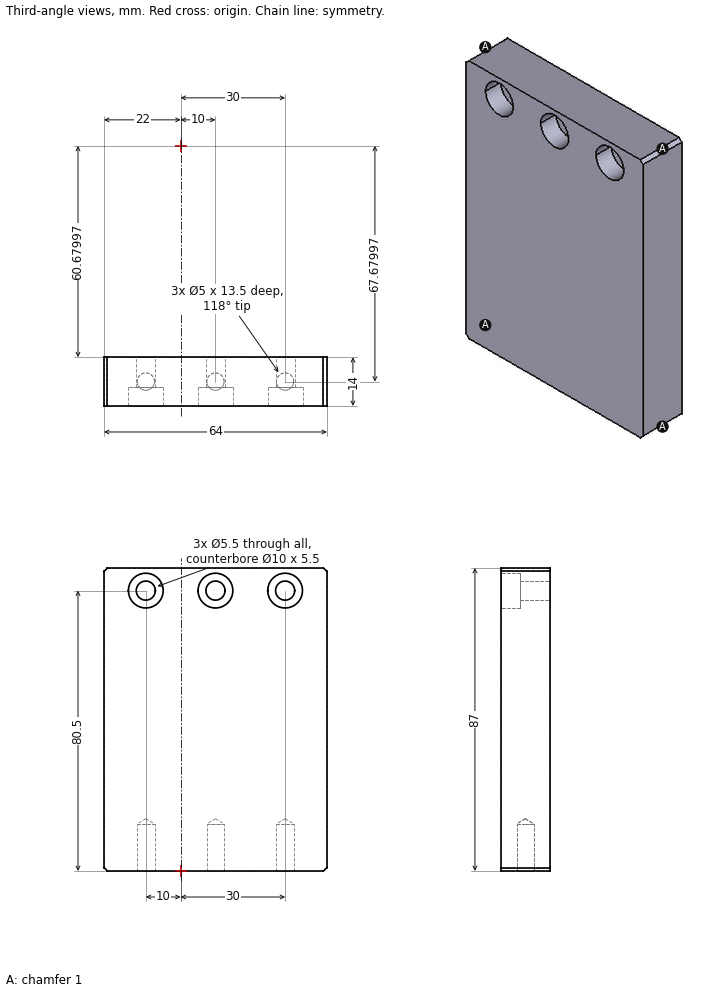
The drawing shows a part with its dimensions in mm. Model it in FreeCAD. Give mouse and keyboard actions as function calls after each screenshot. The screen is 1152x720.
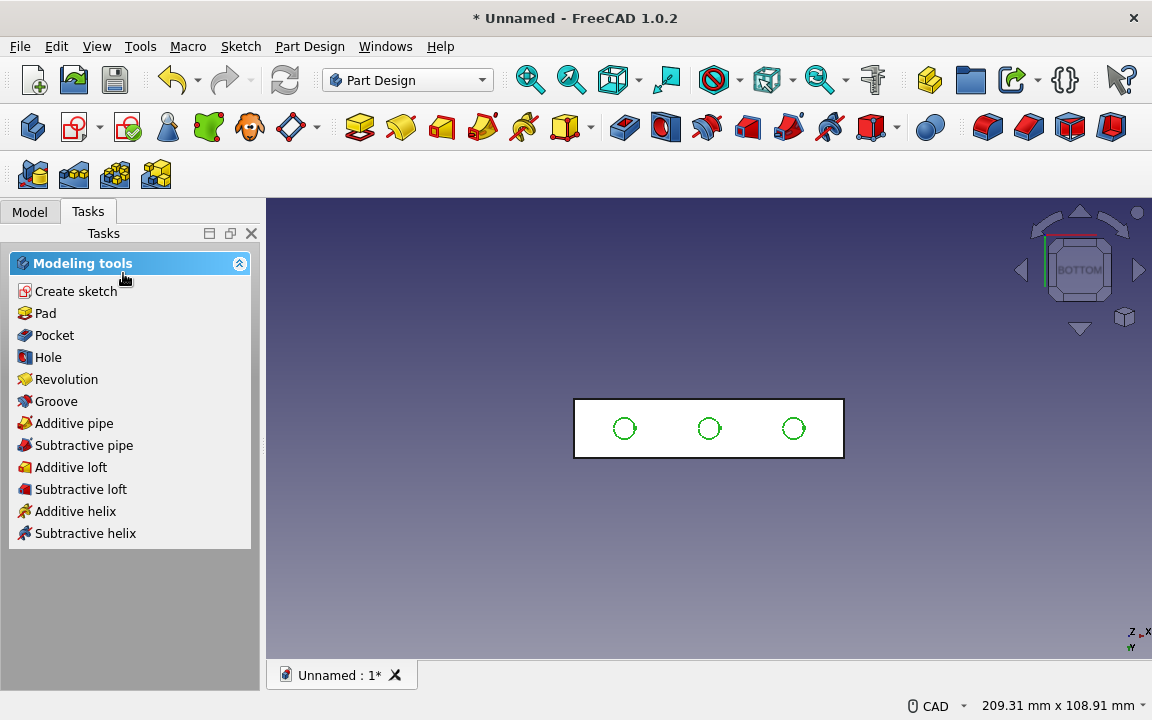
click(666, 128)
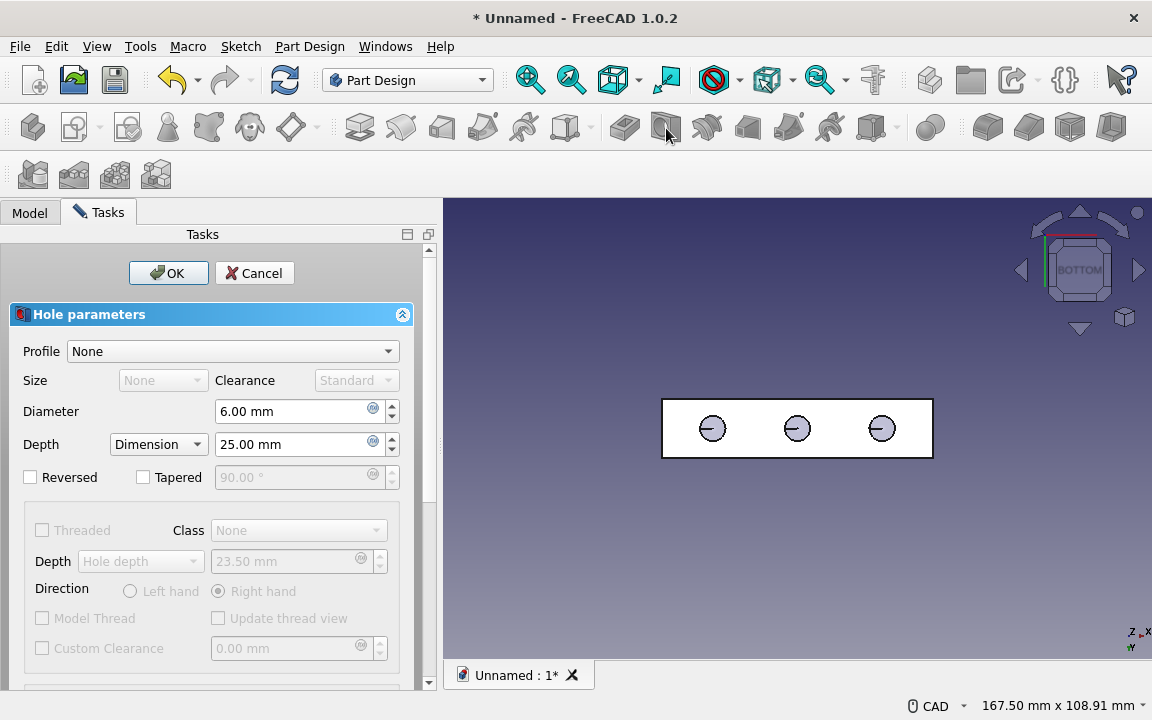
triple_click(300, 412)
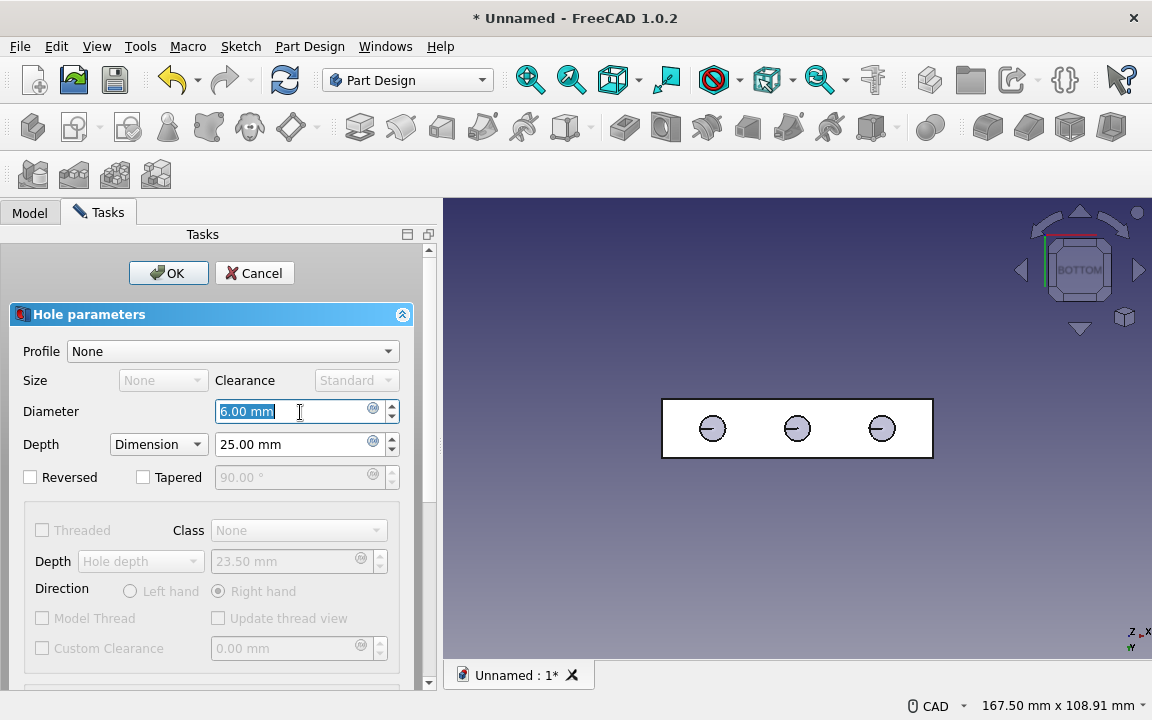
text(5)
key(Tab)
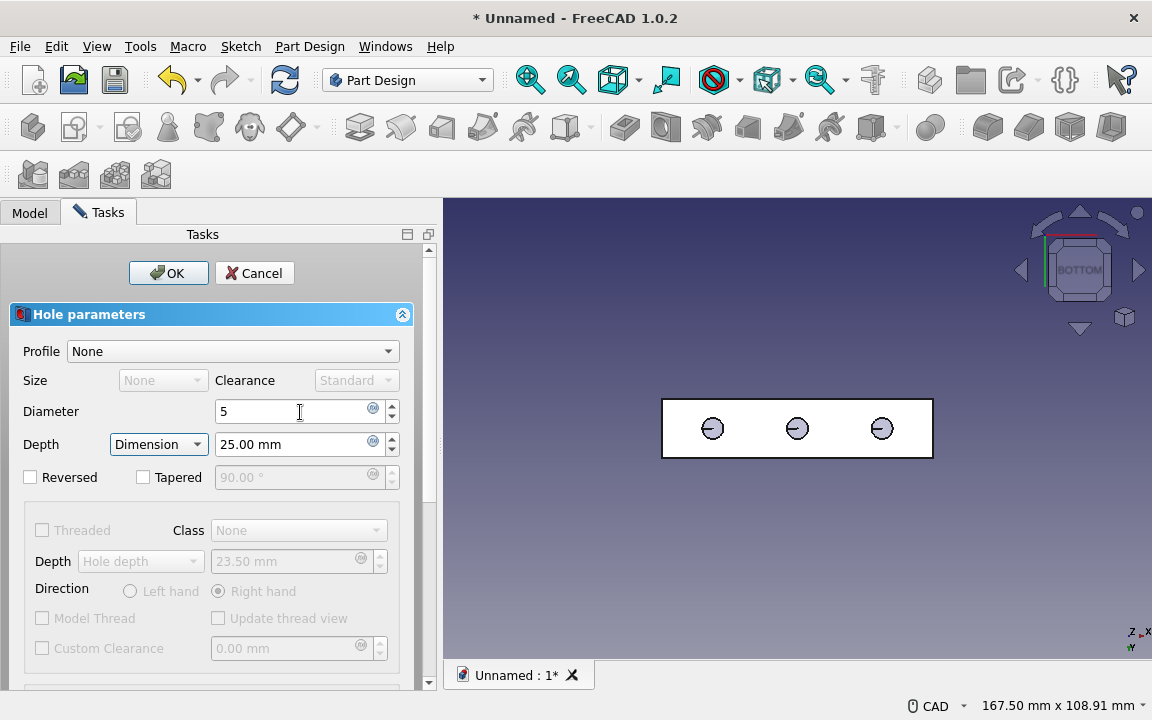
triple_click(300, 444)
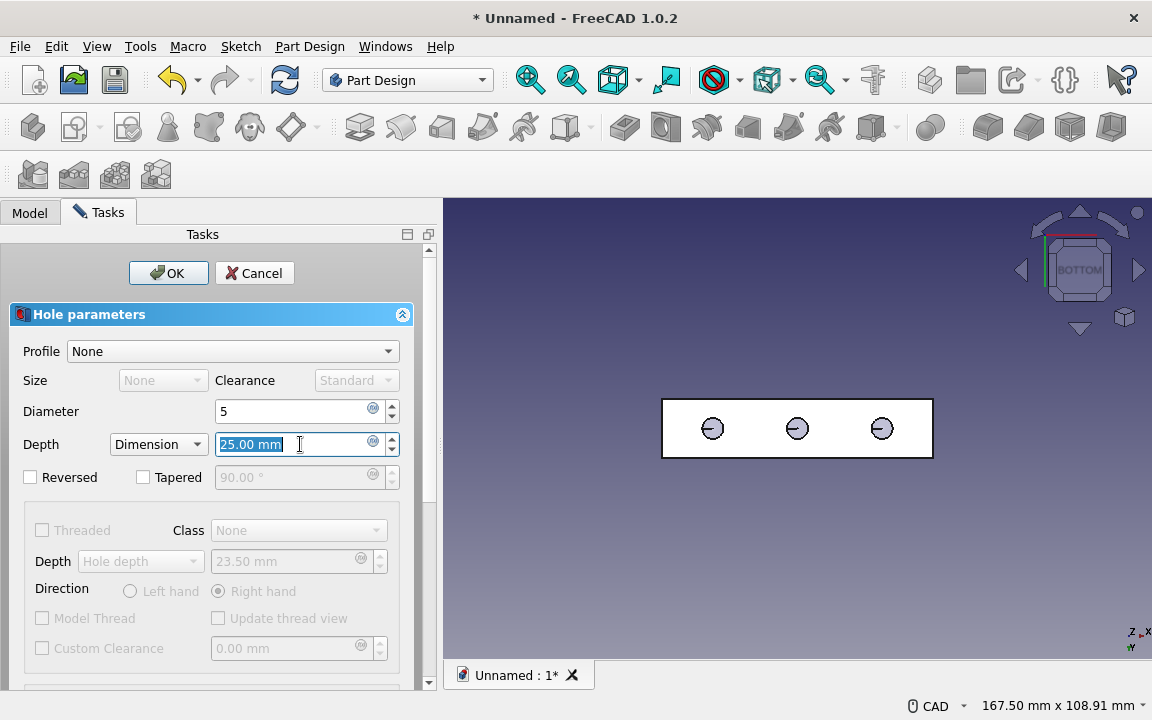
text(13.5)
key(Tab)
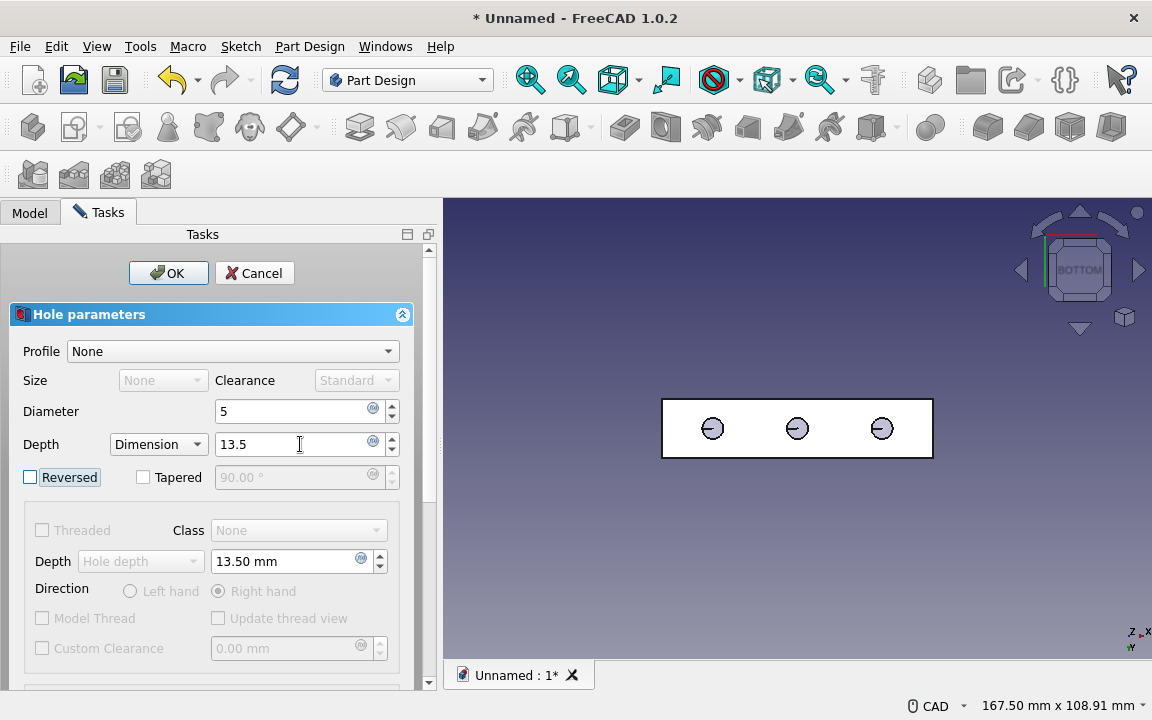
click(169, 273)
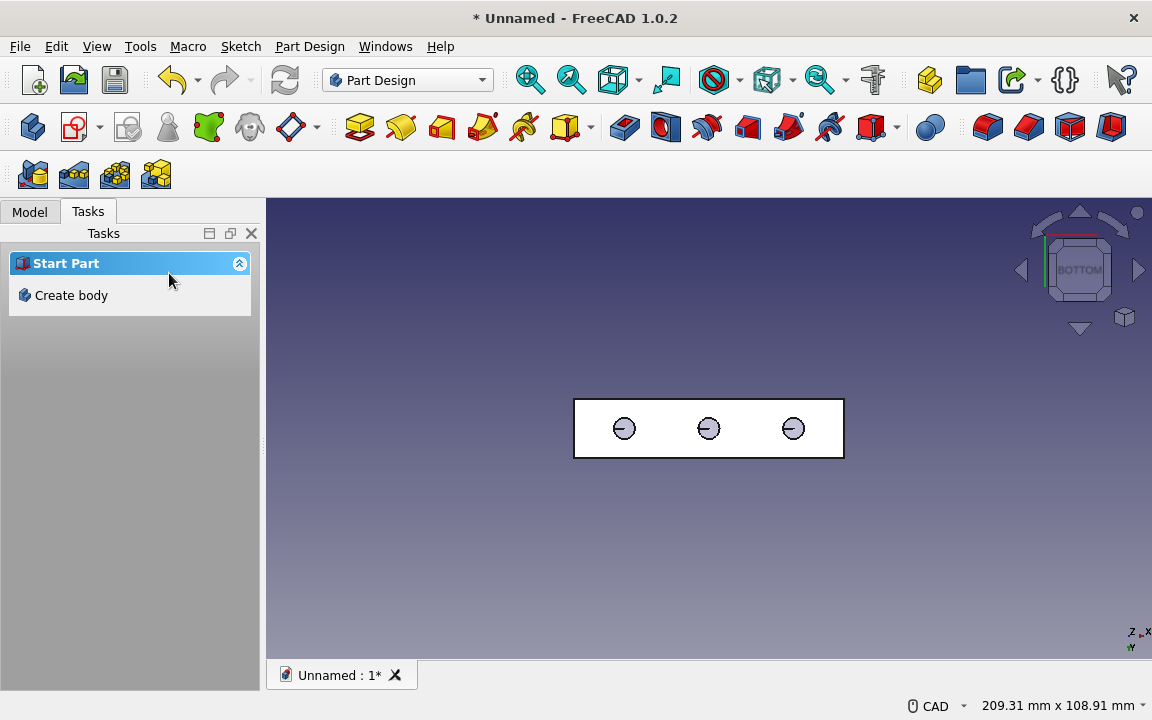
key(v)
key(f)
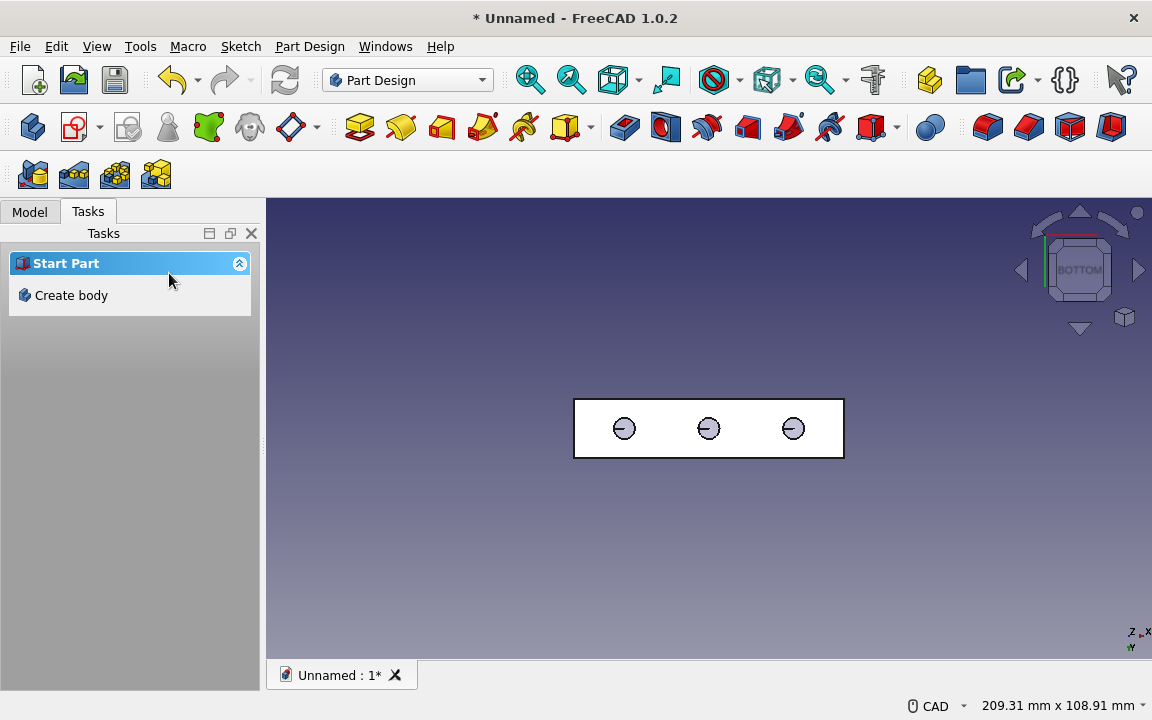
click(844, 427)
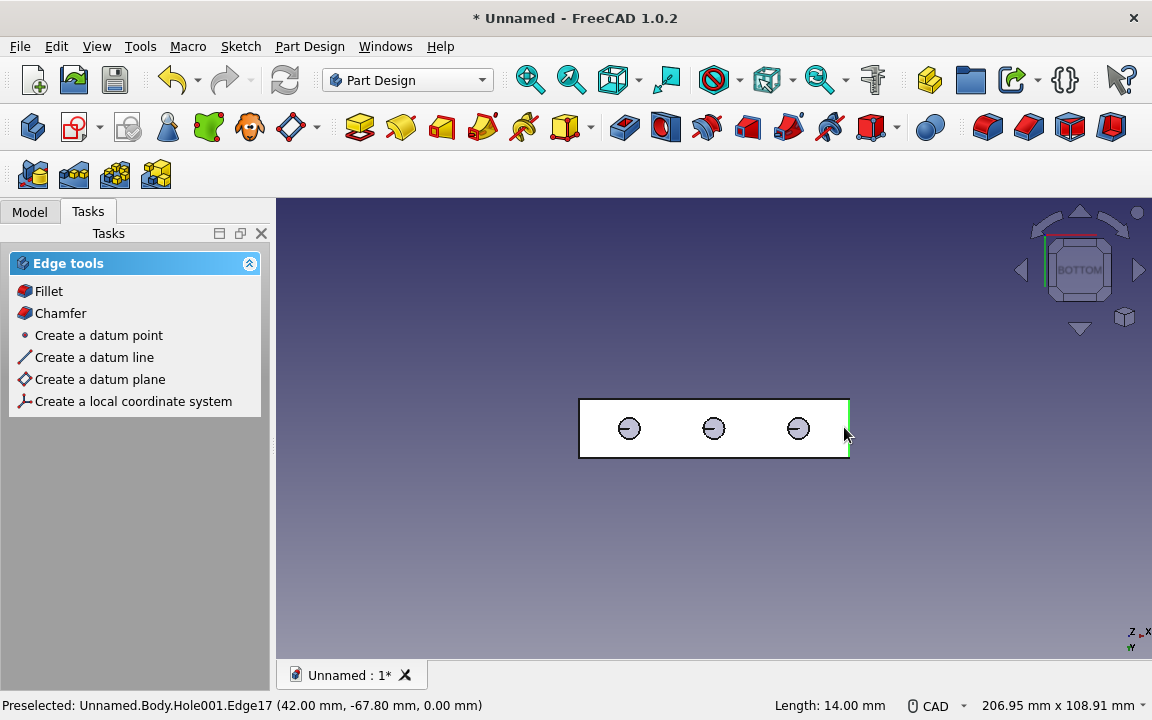
click(579, 427, ctrl)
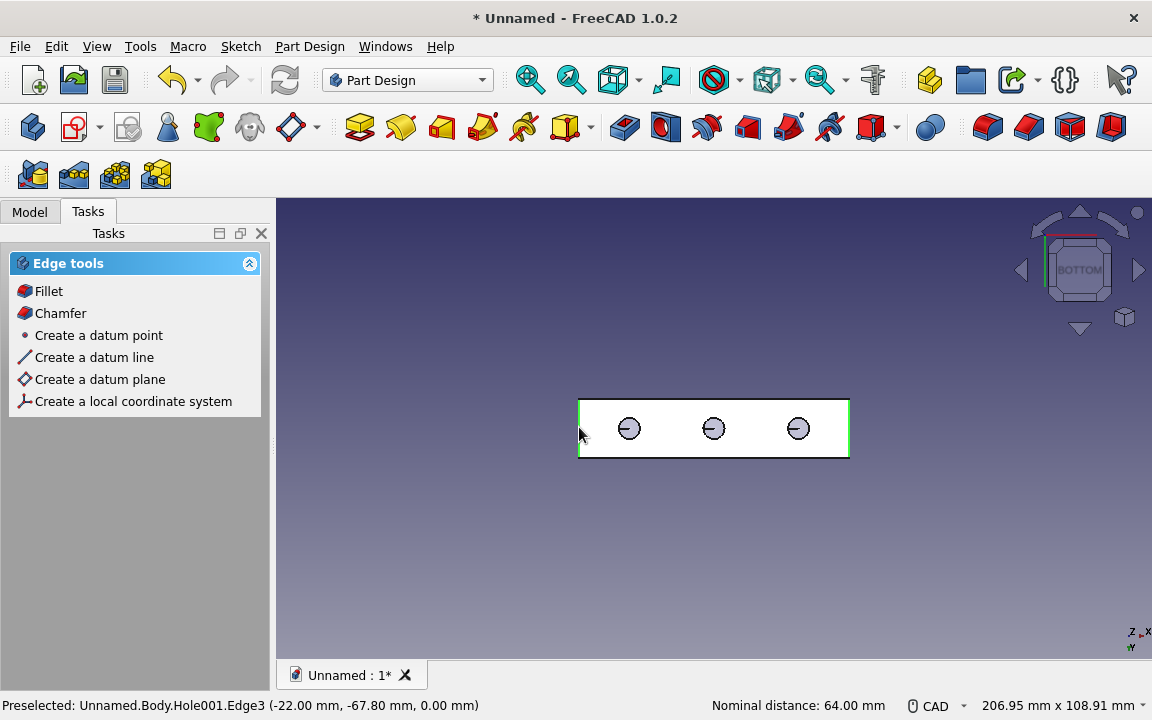
key(0)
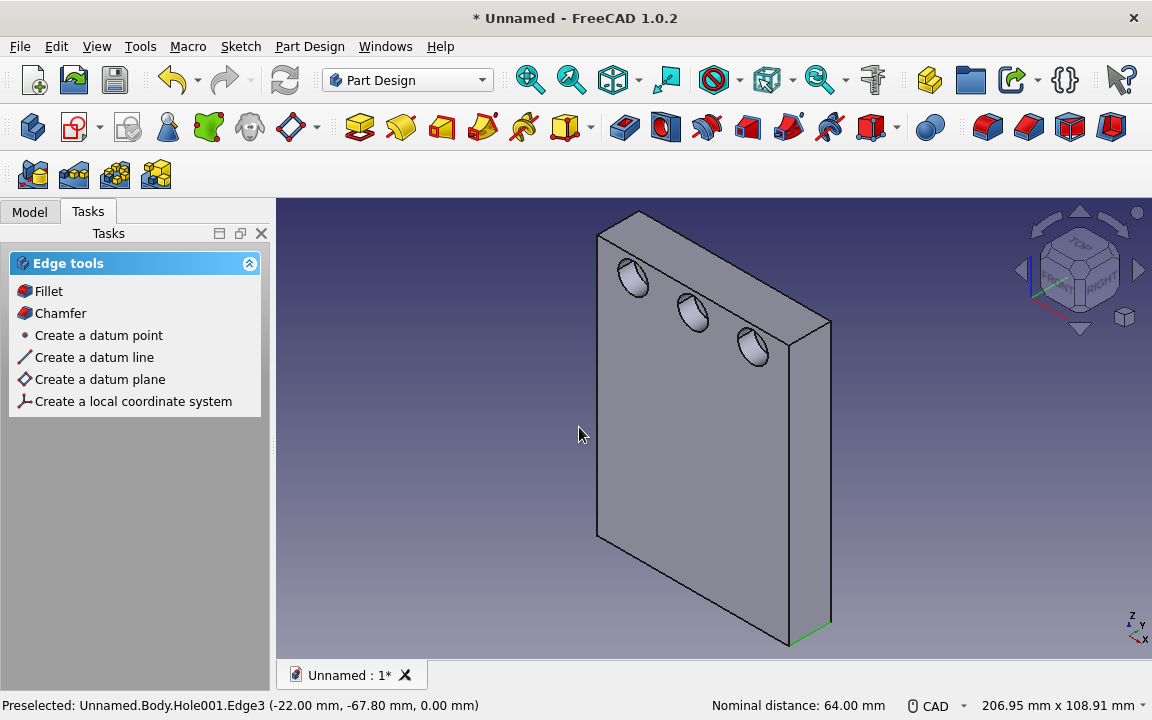
click(810, 332, ctrl)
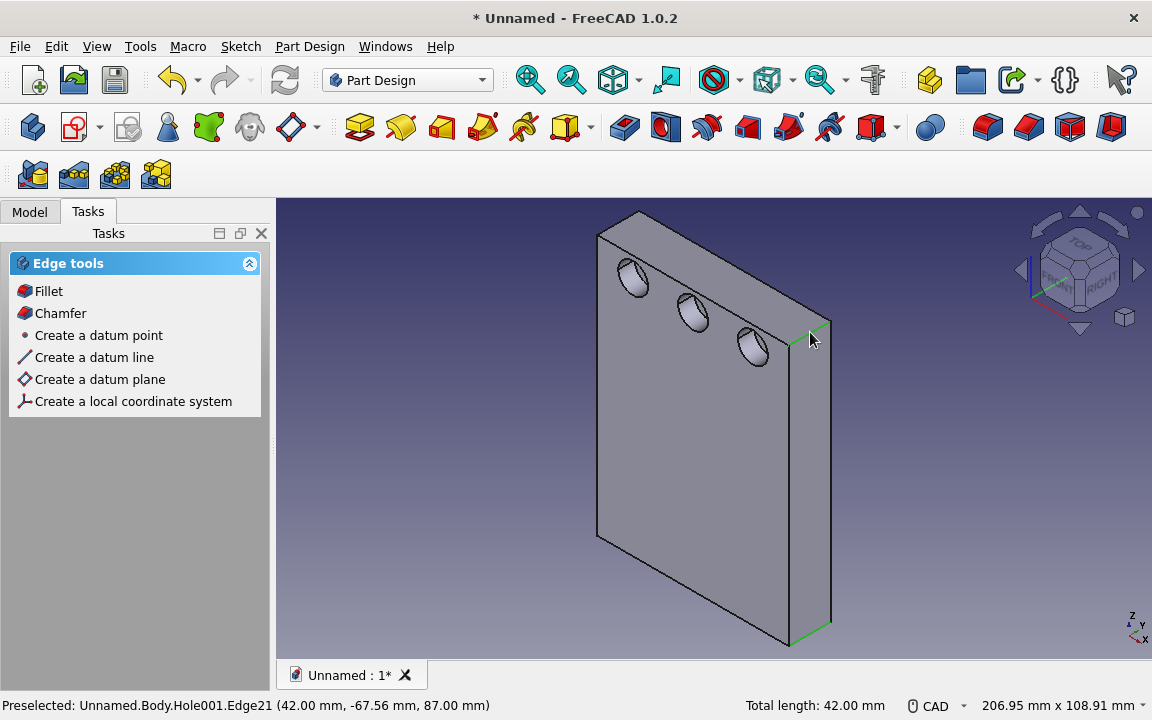
key(2)